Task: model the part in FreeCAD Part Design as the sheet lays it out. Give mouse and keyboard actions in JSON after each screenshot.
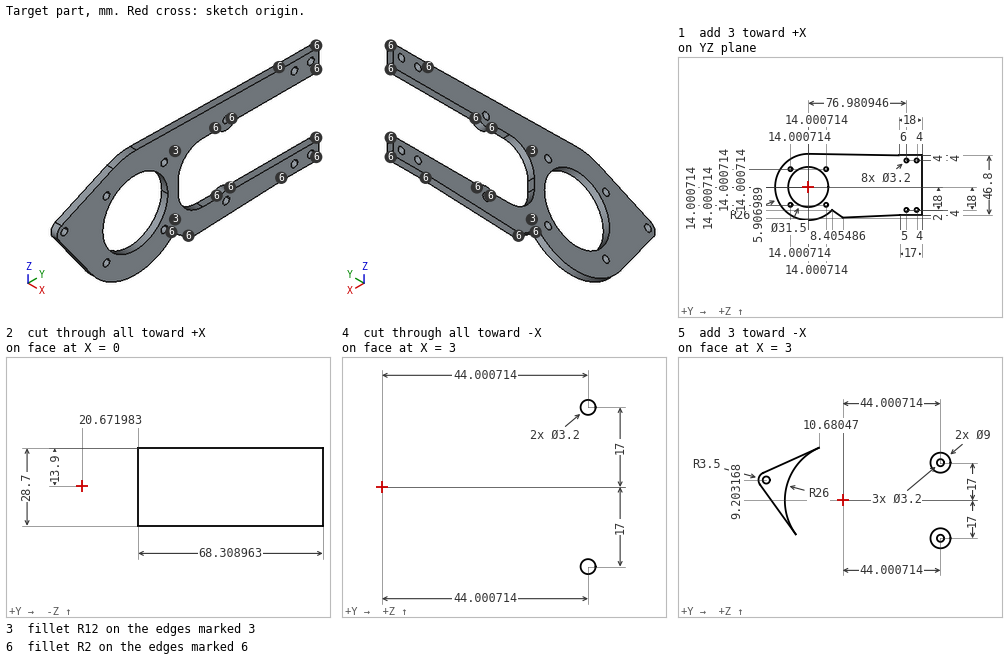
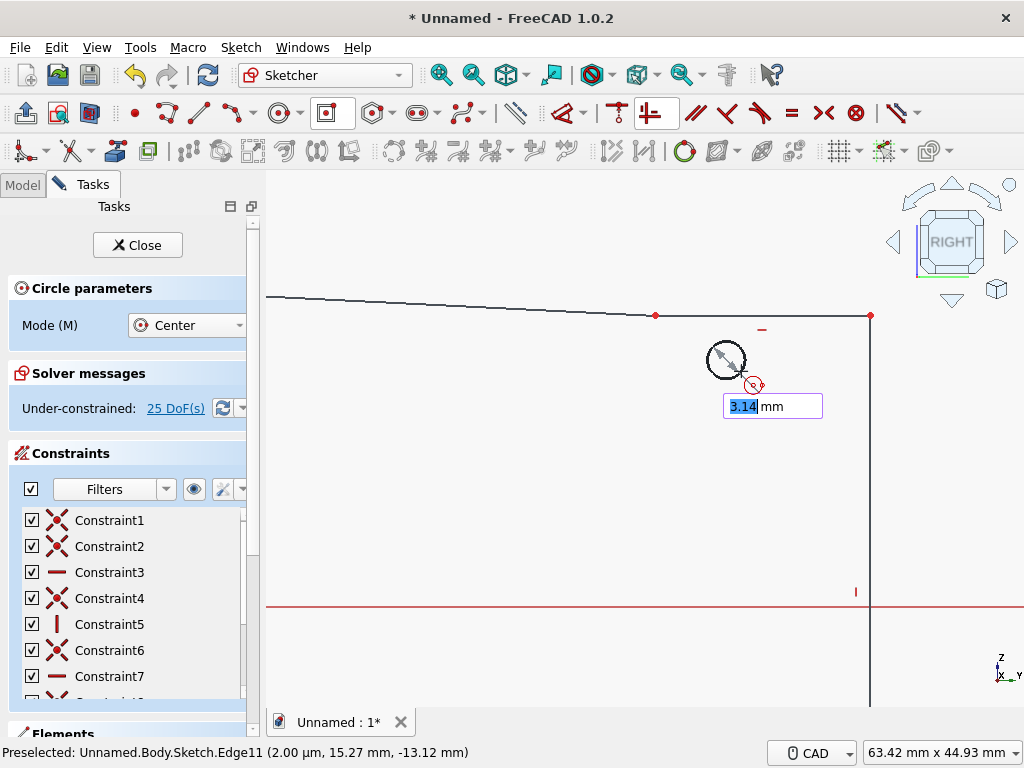
{"action": "left_click", "coordinate": [740, 372]}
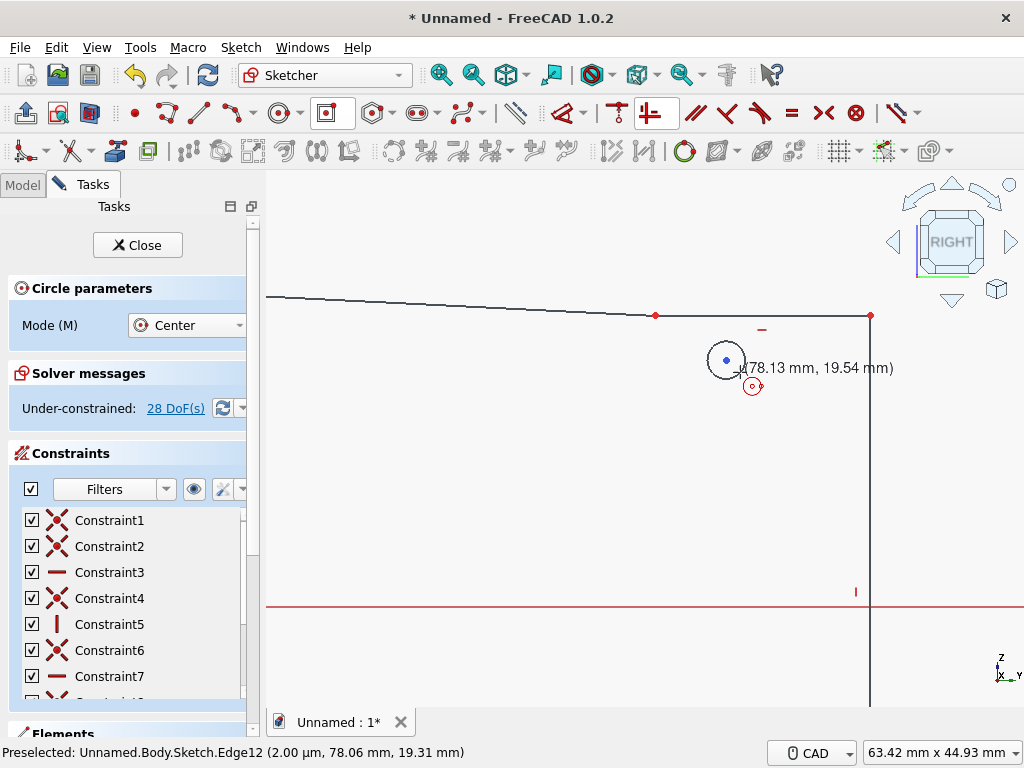
{"action": "scroll", "coordinate": [741, 371], "scroll_direction": "down", "scroll_amount": 6}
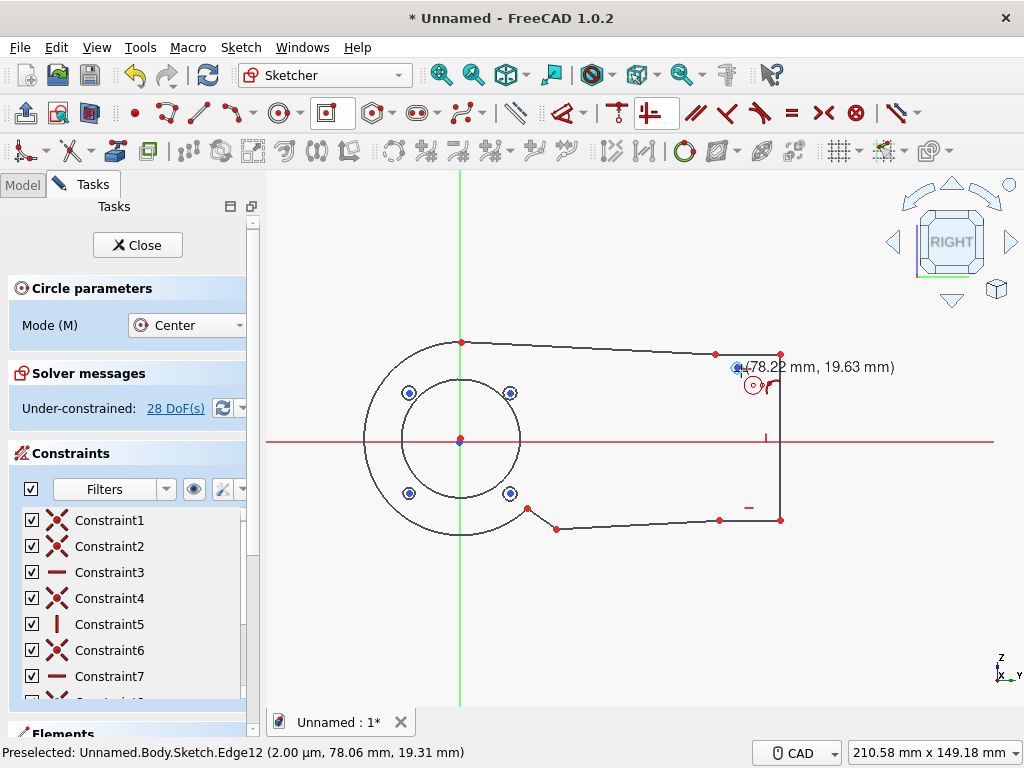
{"action": "left_click", "coordinate": [766, 367]}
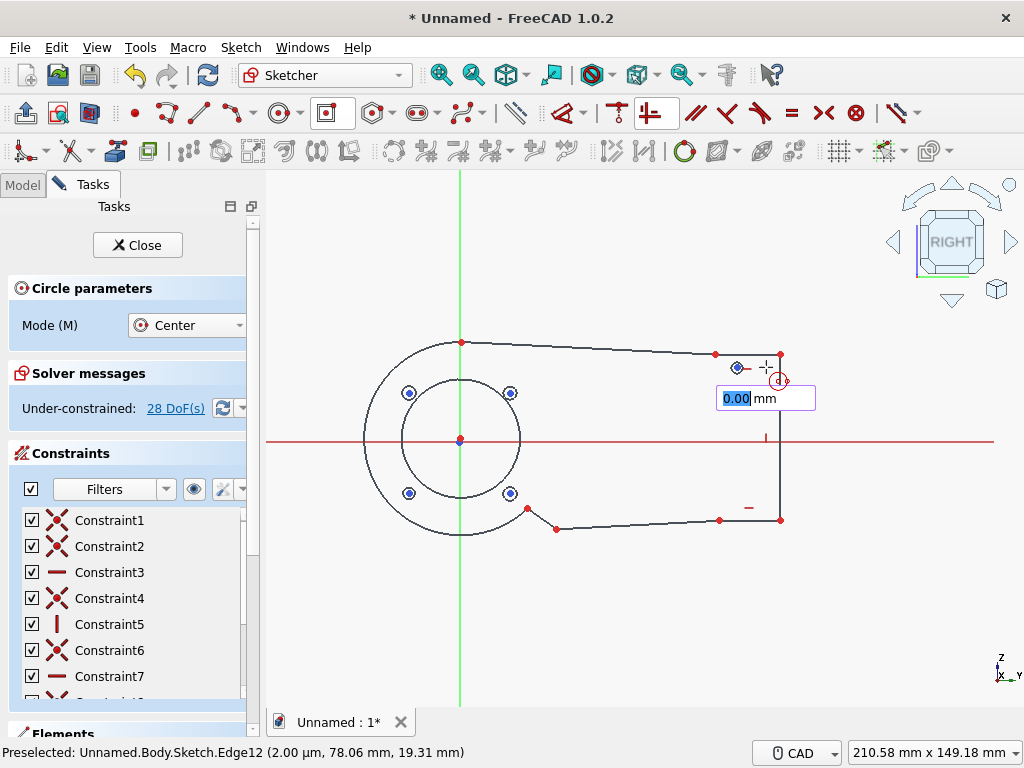
{"action": "scroll", "coordinate": [762, 371], "scroll_direction": "up", "scroll_amount": 6}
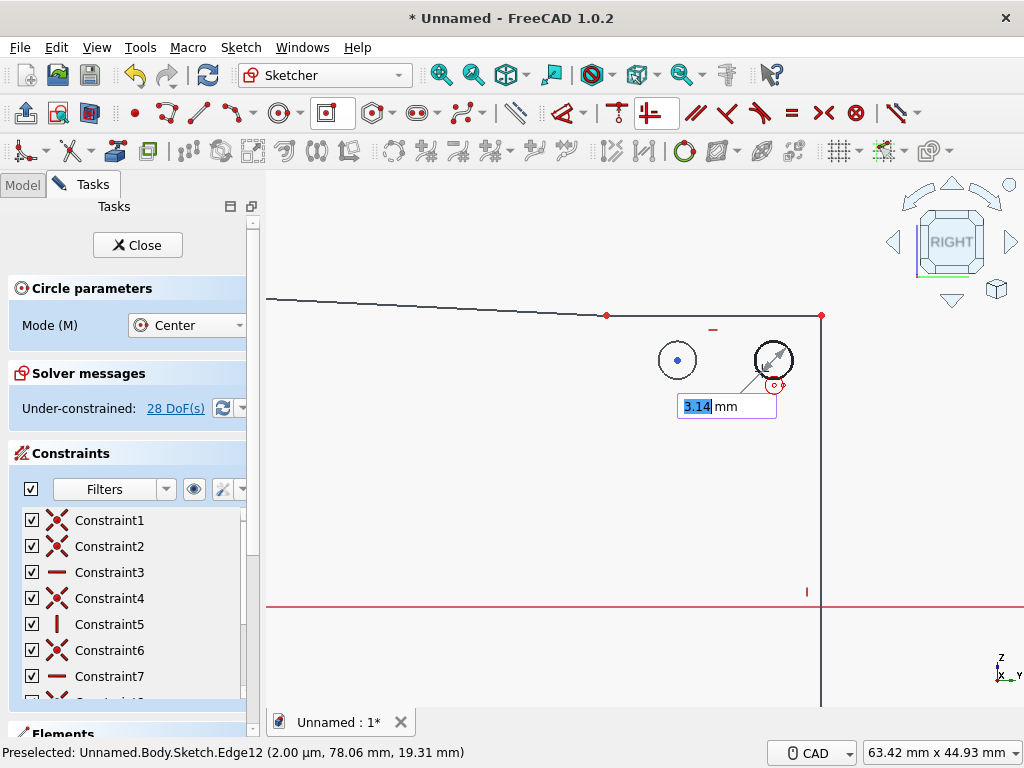
{"action": "left_click", "coordinate": [760, 372]}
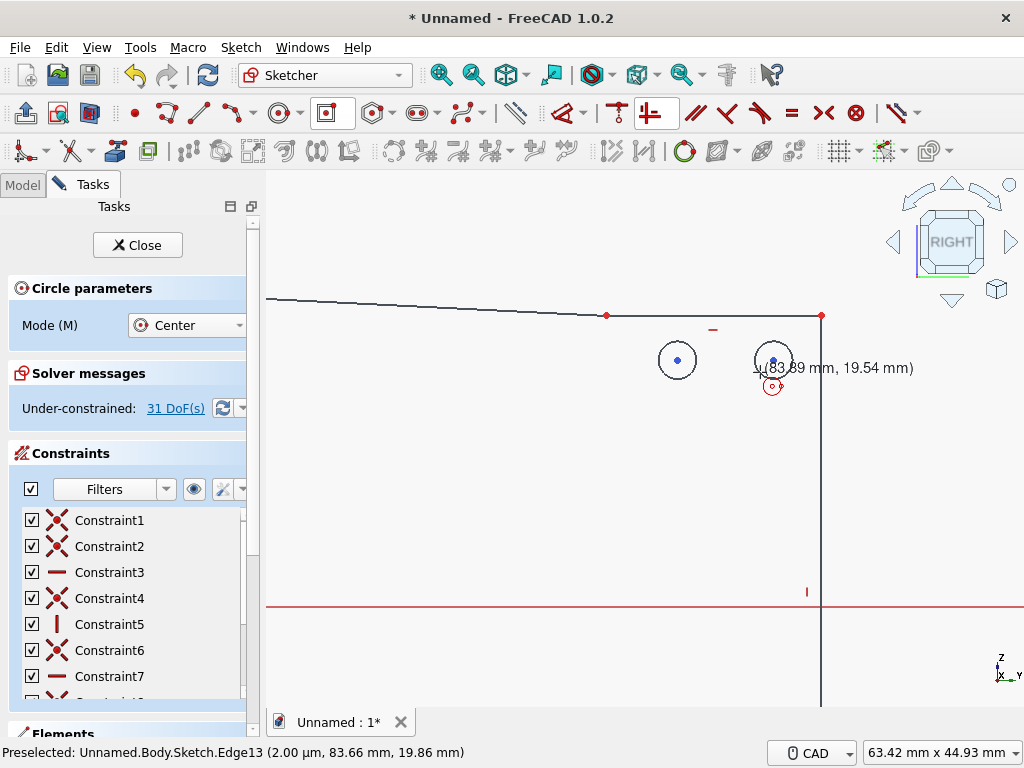
{"action": "scroll", "coordinate": [762, 371], "scroll_direction": "down", "scroll_amount": 6}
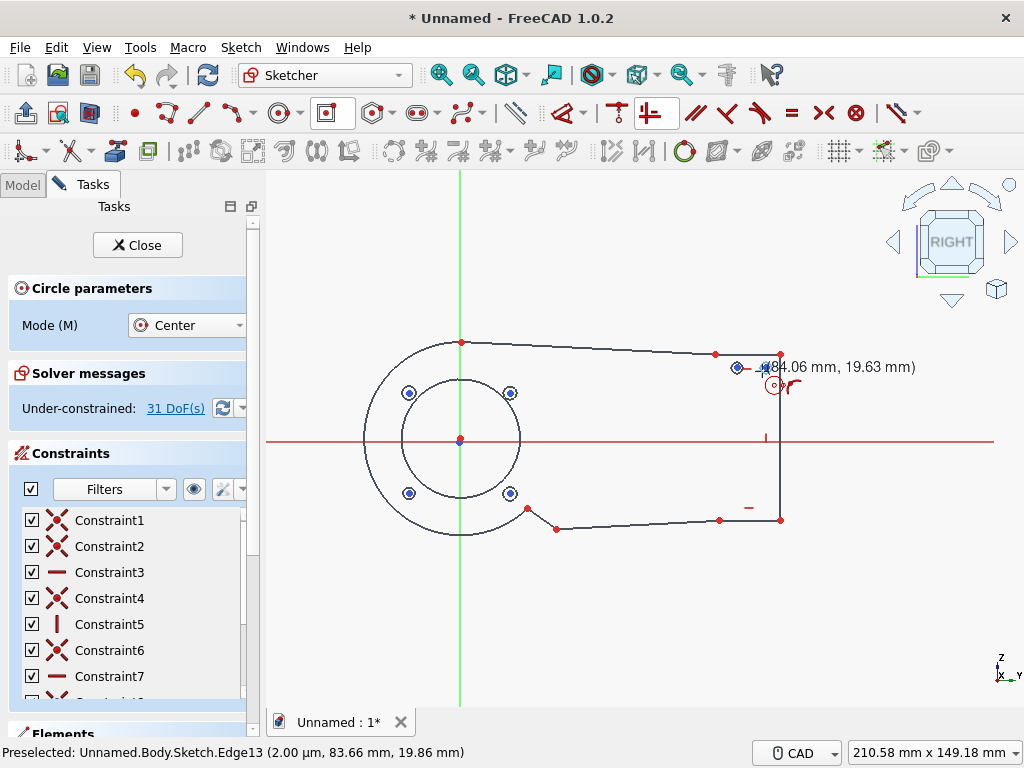
{"action": "scroll", "coordinate": [737, 507], "scroll_direction": "up", "scroll_amount": 7}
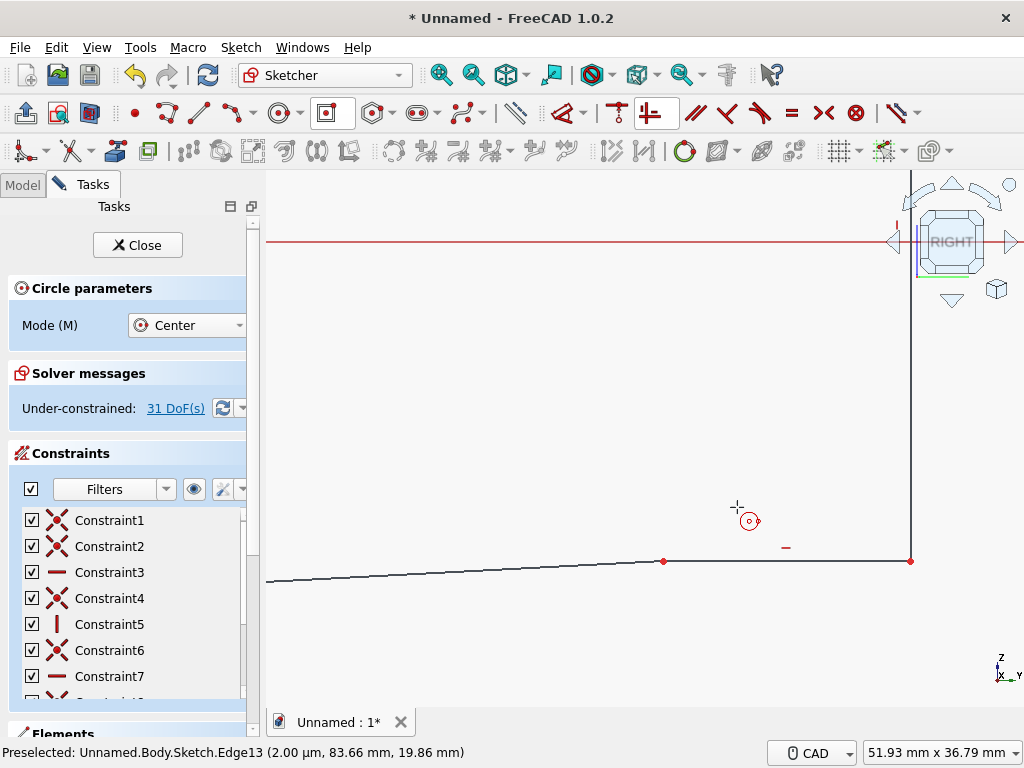
{"action": "scroll", "coordinate": [737, 507], "scroll_direction": "down", "scroll_amount": 7}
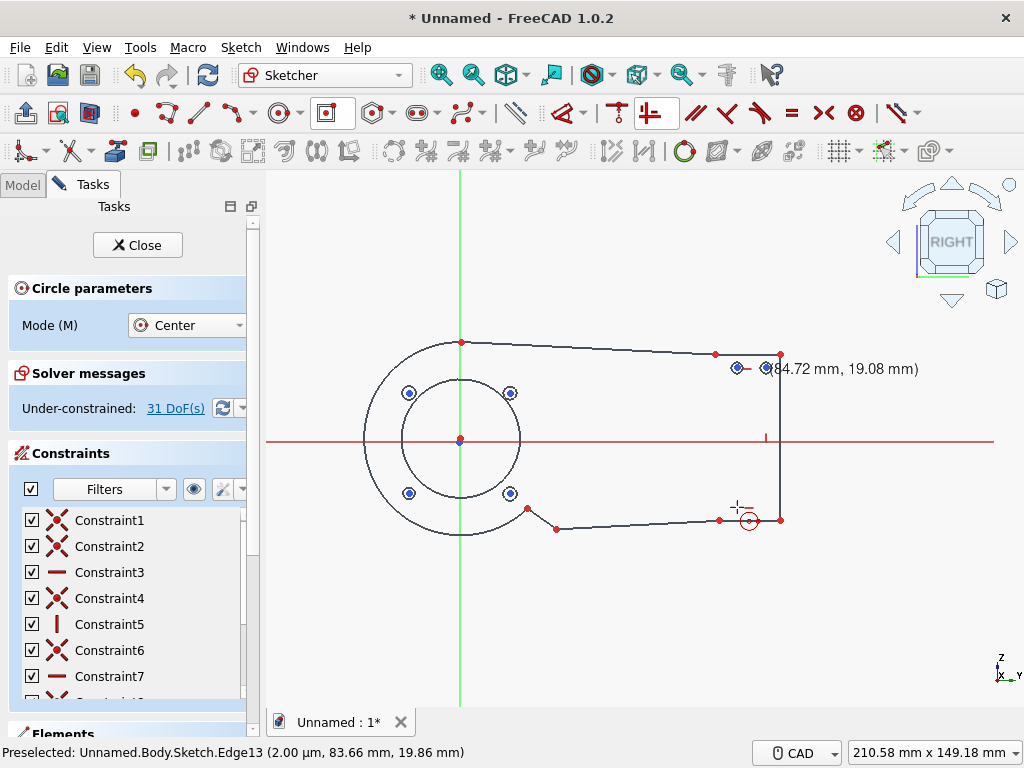
{"action": "left_click", "coordinate": [737, 507]}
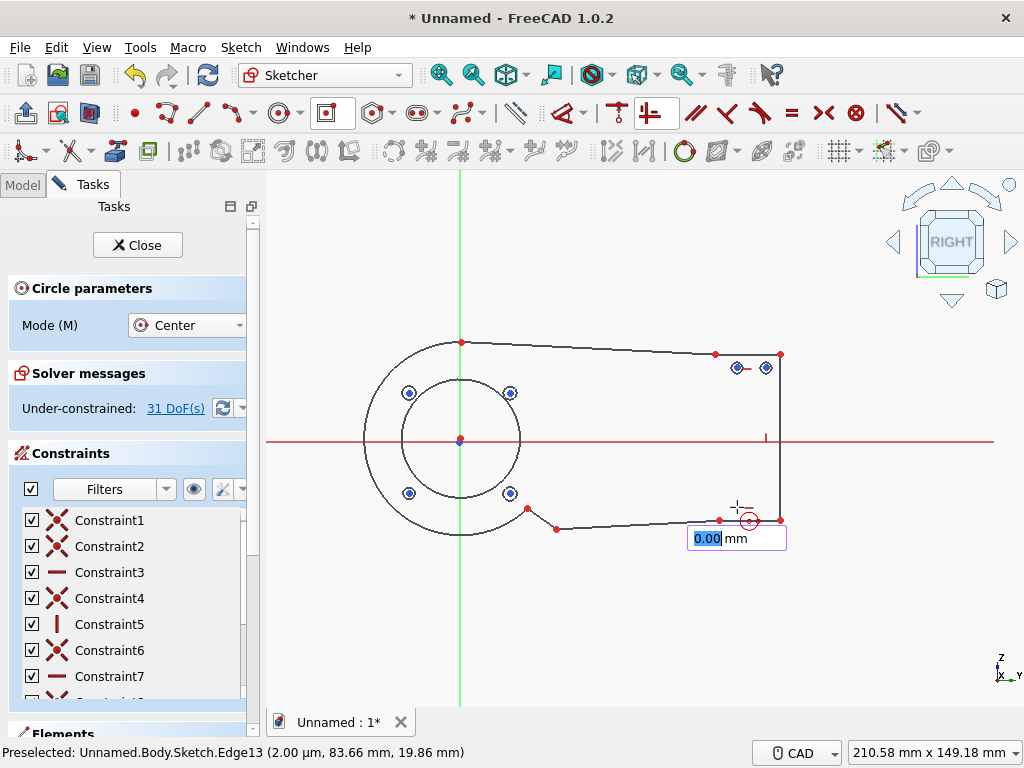
{"action": "scroll", "coordinate": [741, 503], "scroll_direction": "up", "scroll_amount": 6}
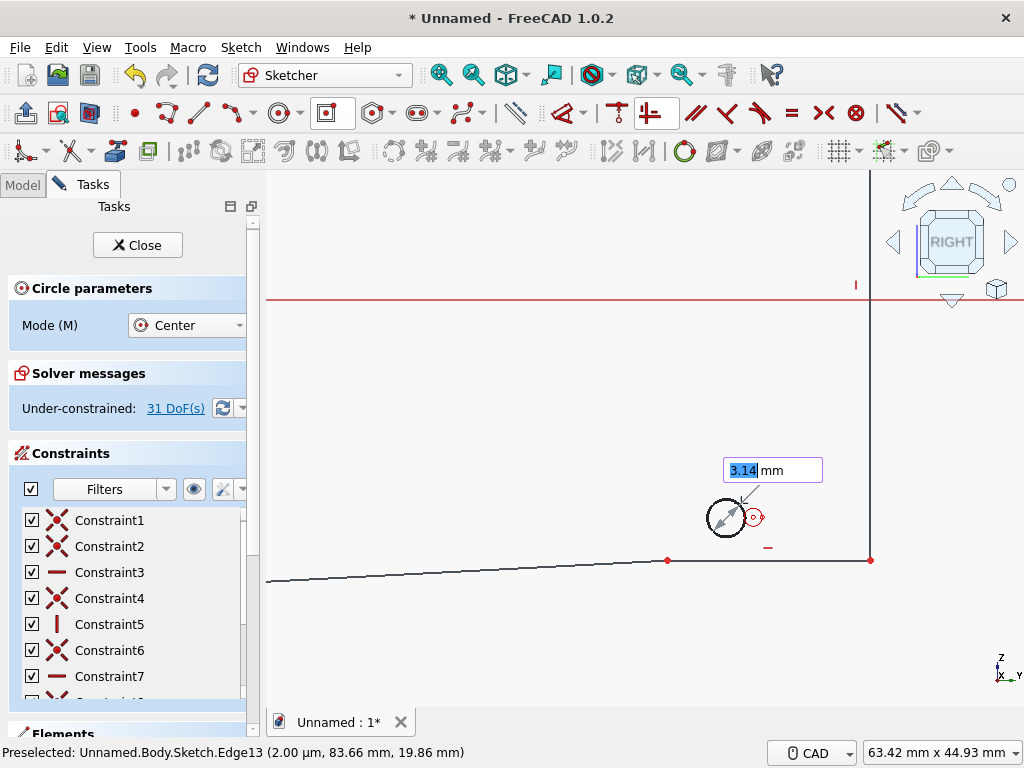
{"action": "left_click", "coordinate": [740, 501]}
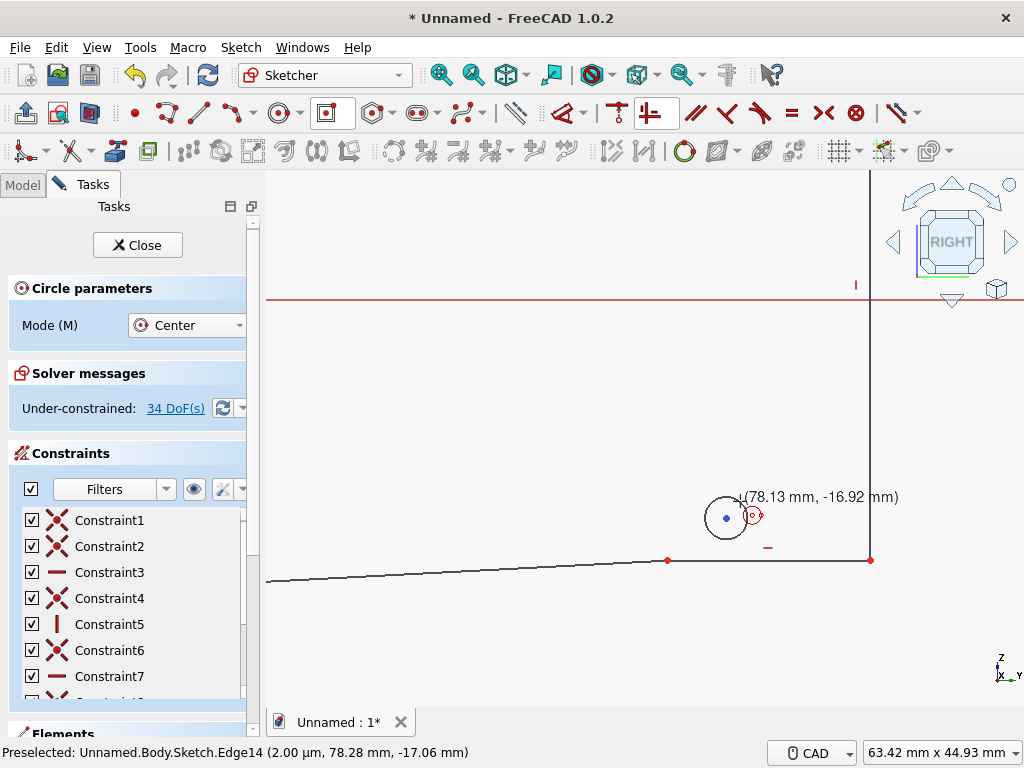
{"action": "scroll", "coordinate": [741, 503], "scroll_direction": "down", "scroll_amount": 6}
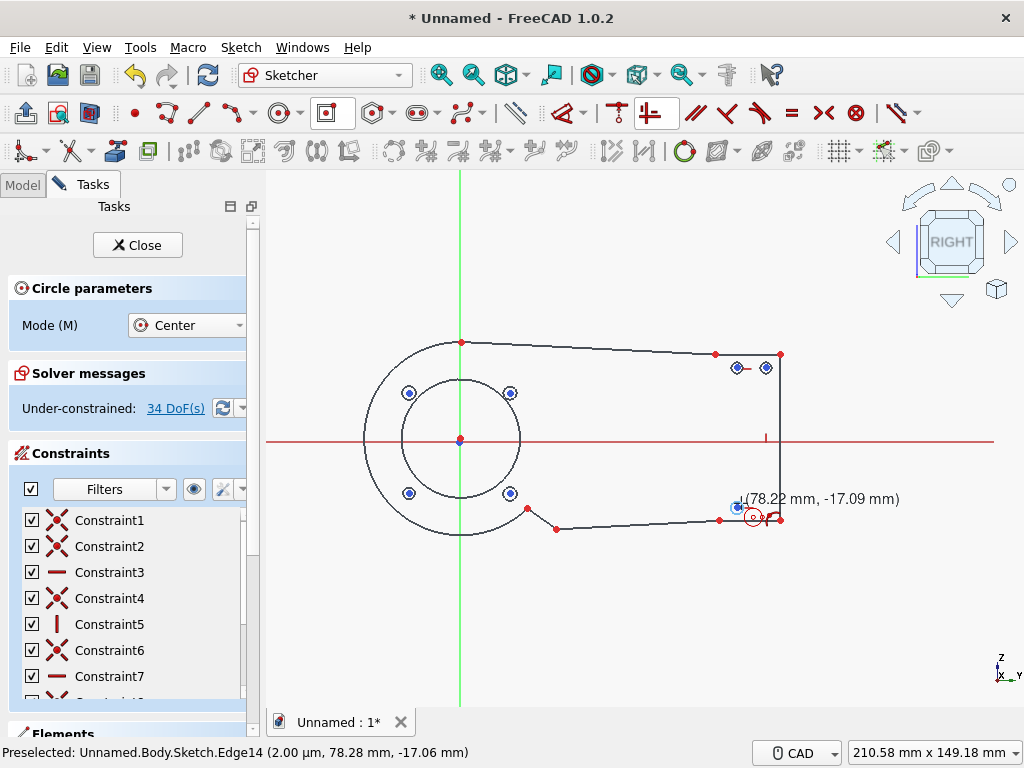
{"action": "left_click", "coordinate": [766, 507]}